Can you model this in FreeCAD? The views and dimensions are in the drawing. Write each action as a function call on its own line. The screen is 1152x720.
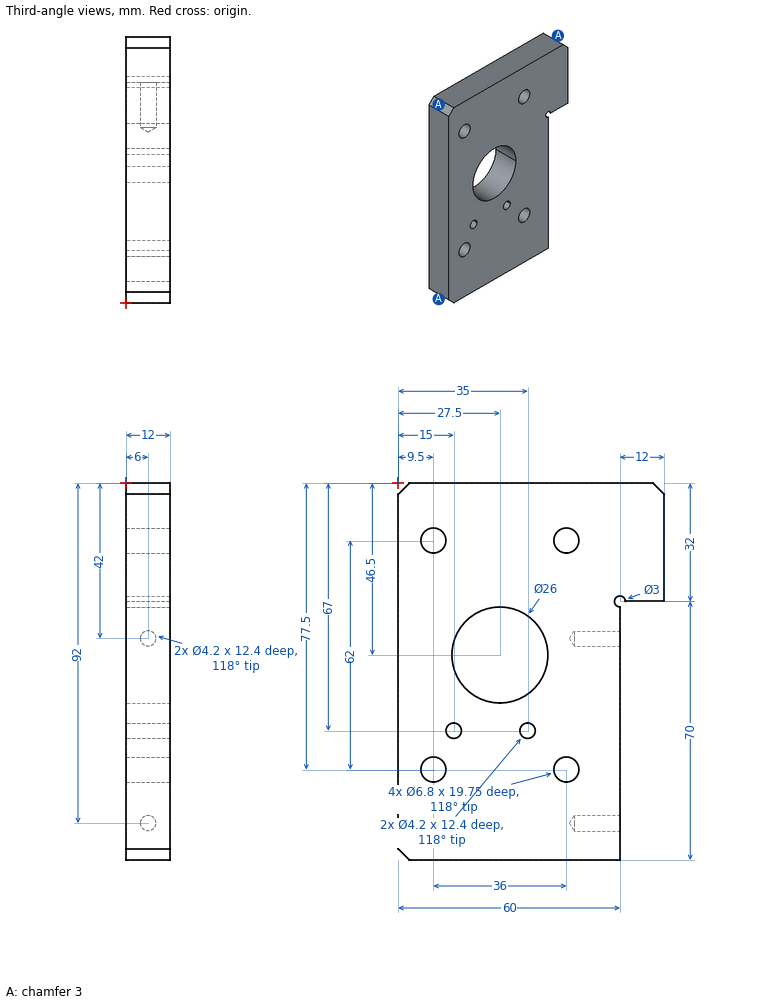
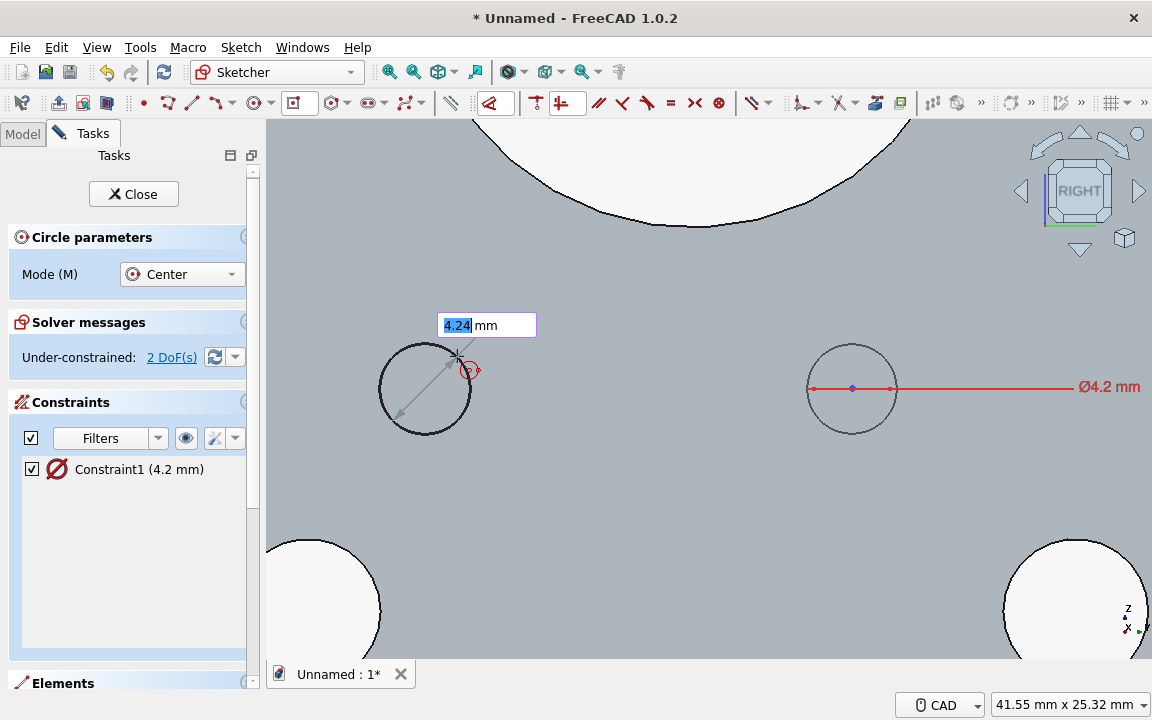
text(4.2)
key(Return)
key(Escape)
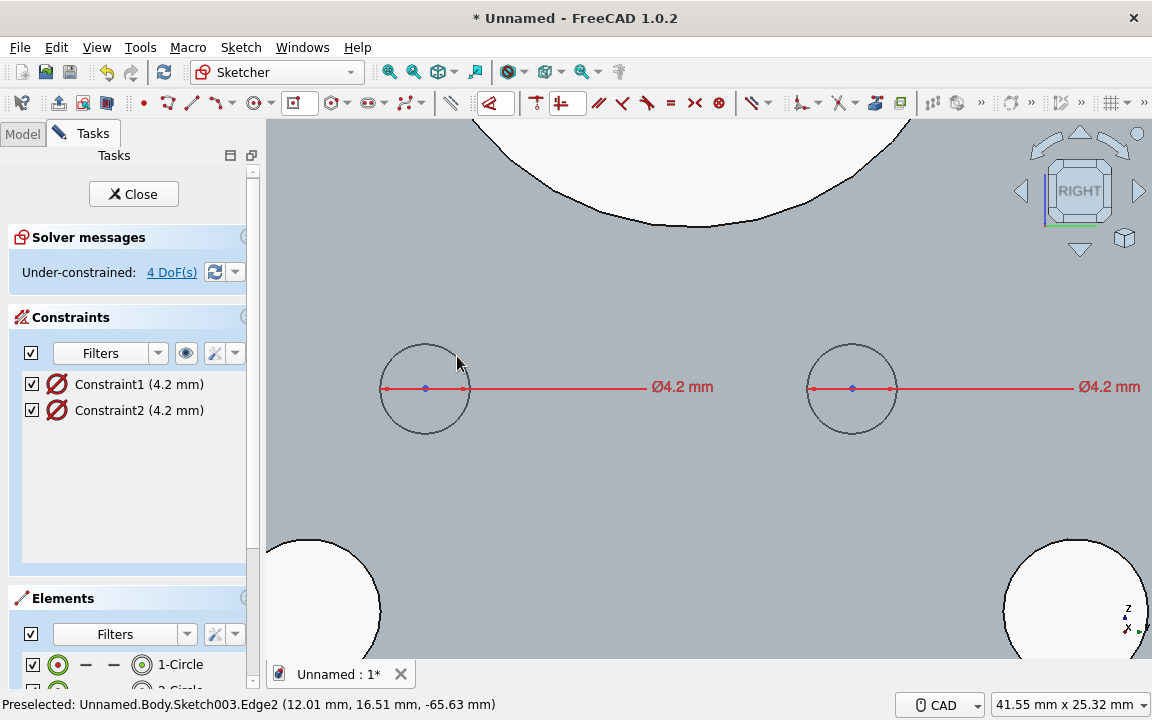
click(852, 389)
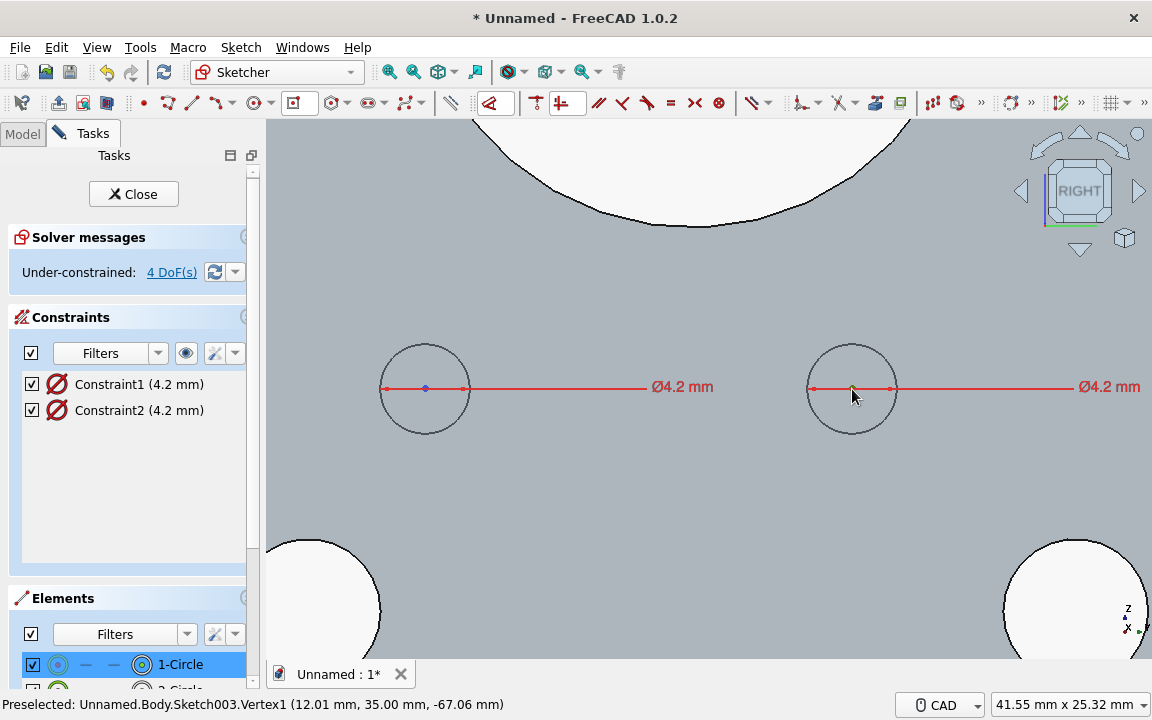
click(425, 389)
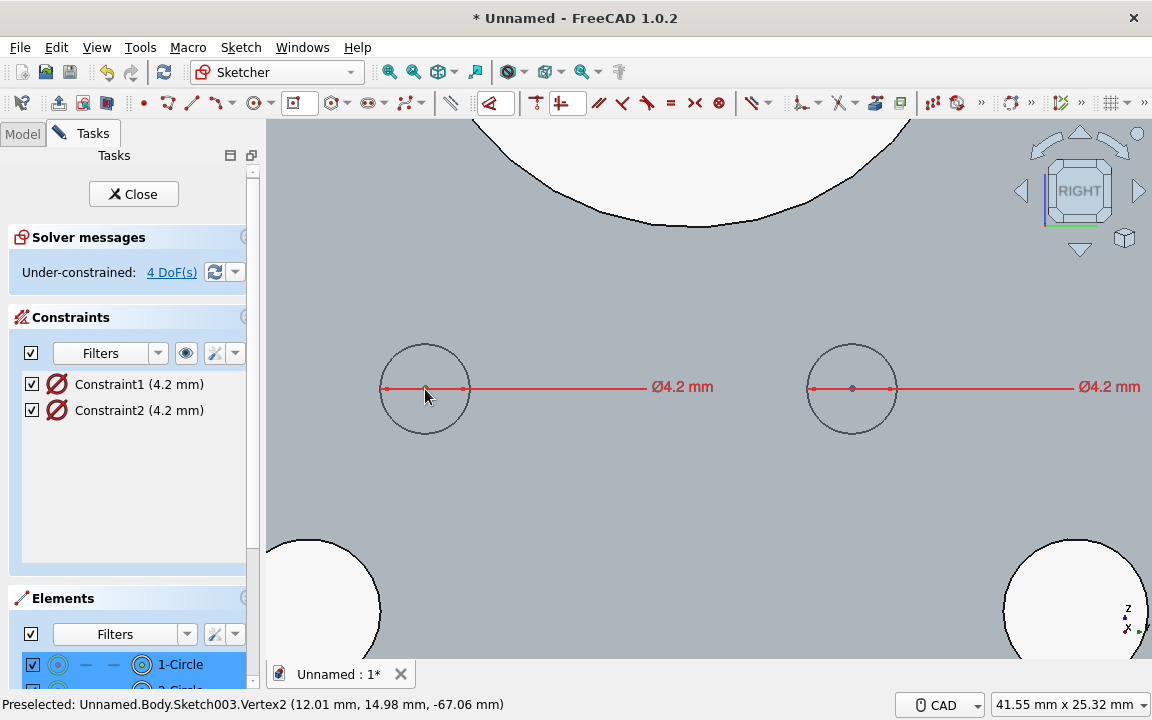
click(580, 104)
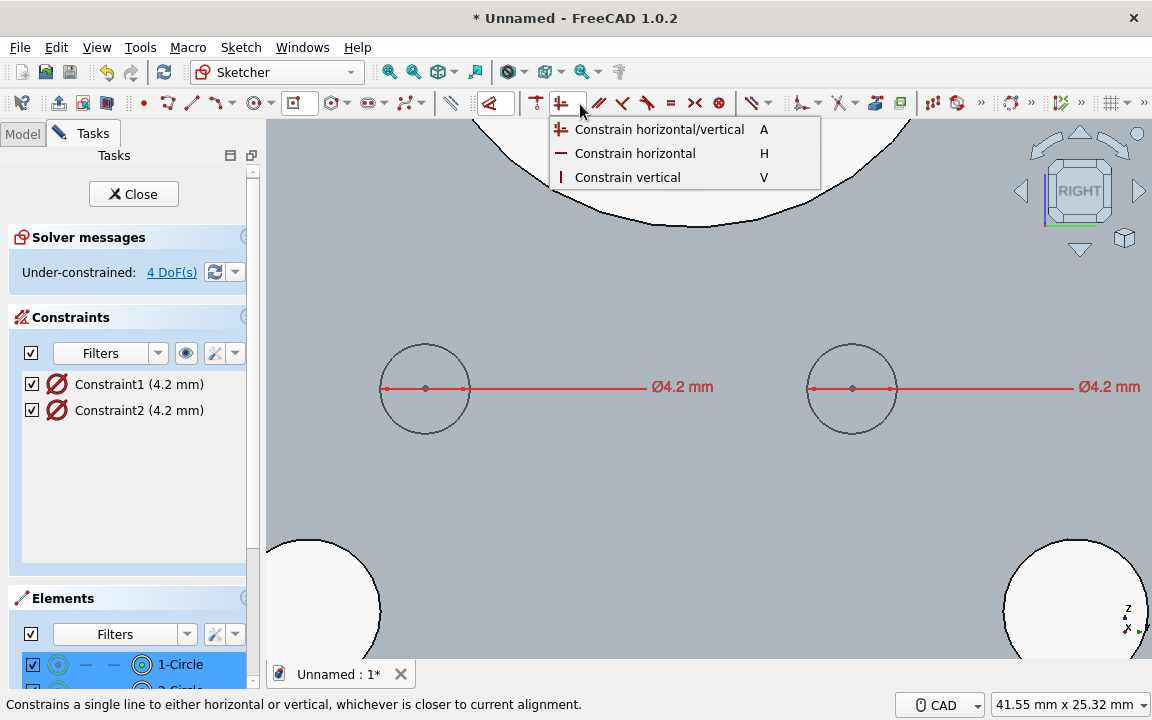
click(685, 153)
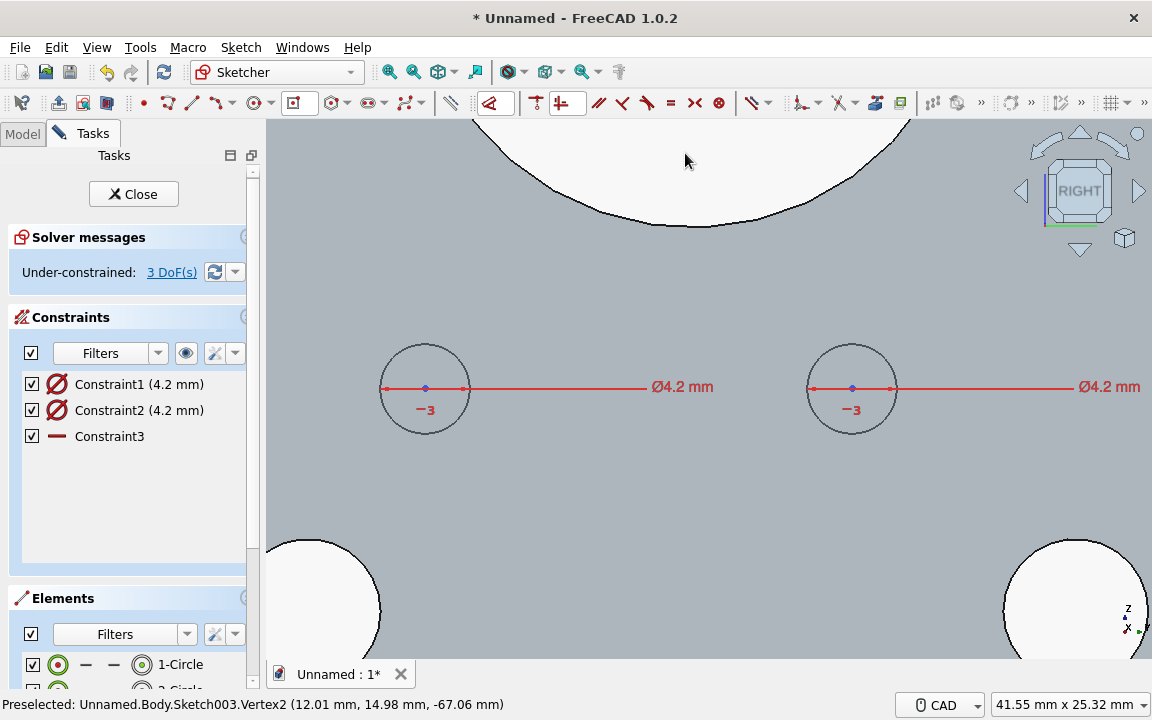
click(852, 389)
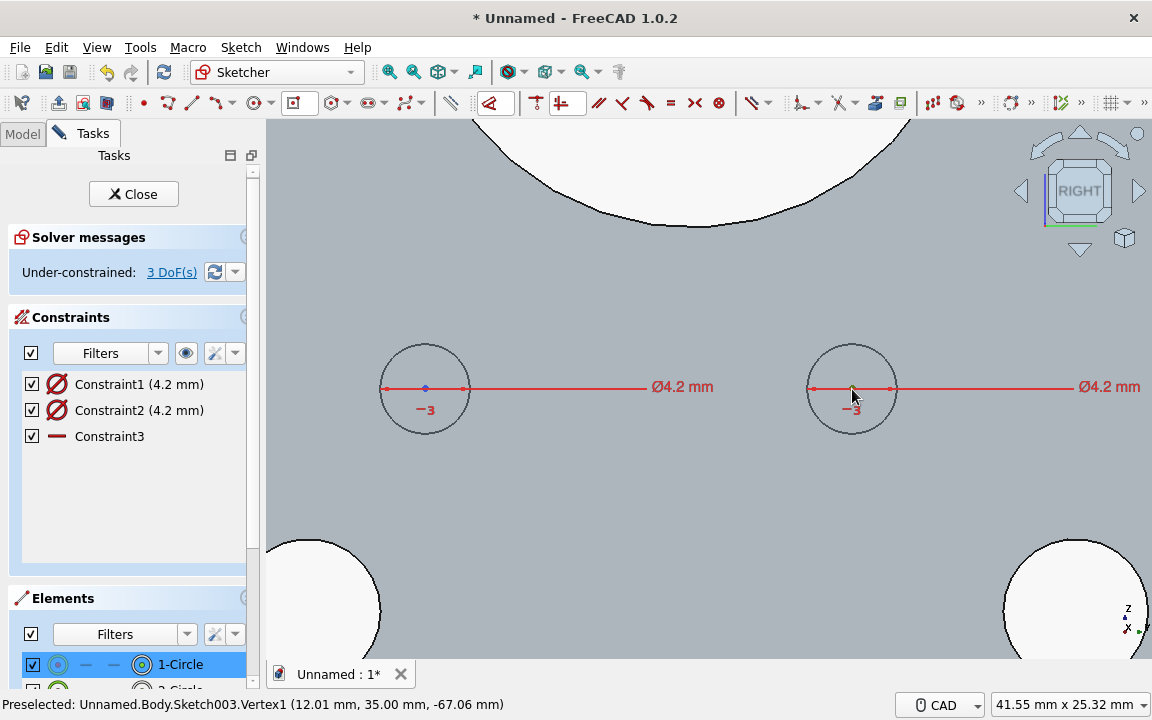
key(l)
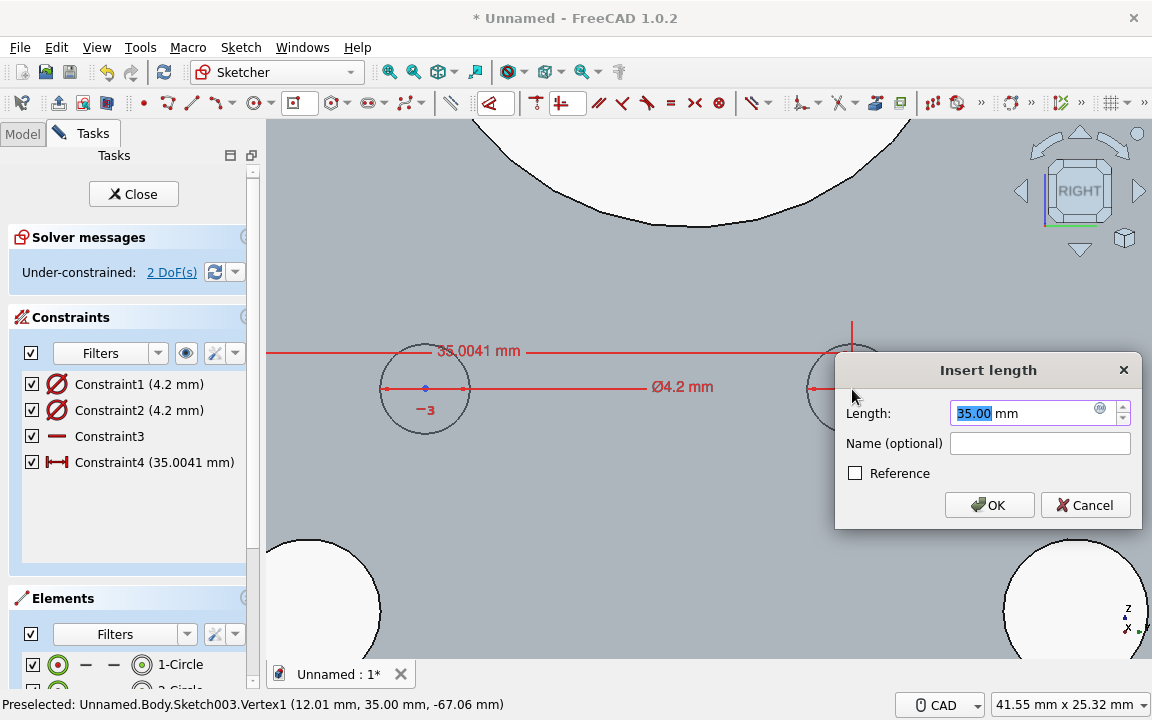
text(35)
key(Return)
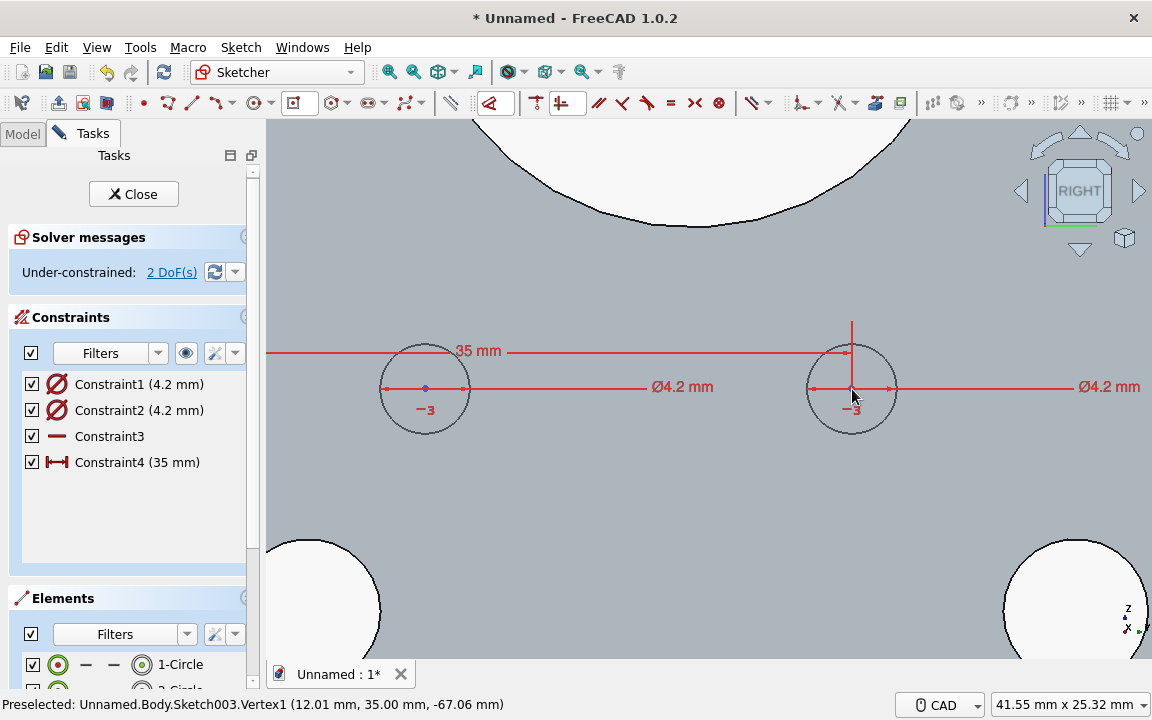
click(852, 389)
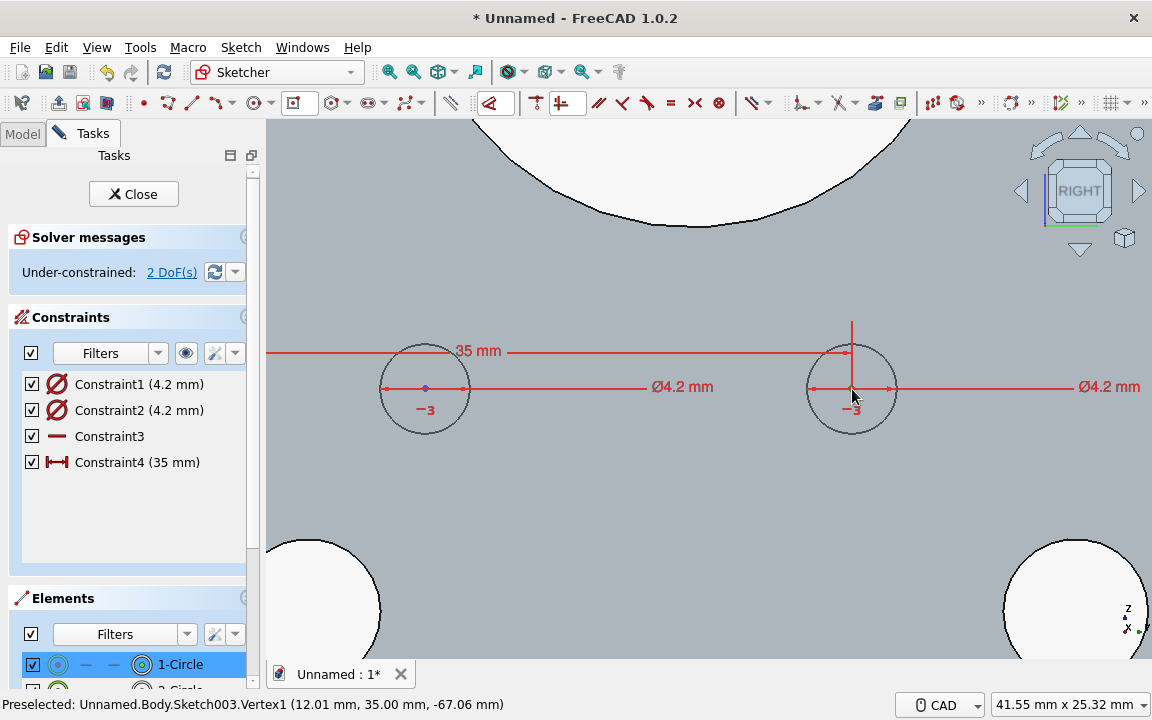
key(i)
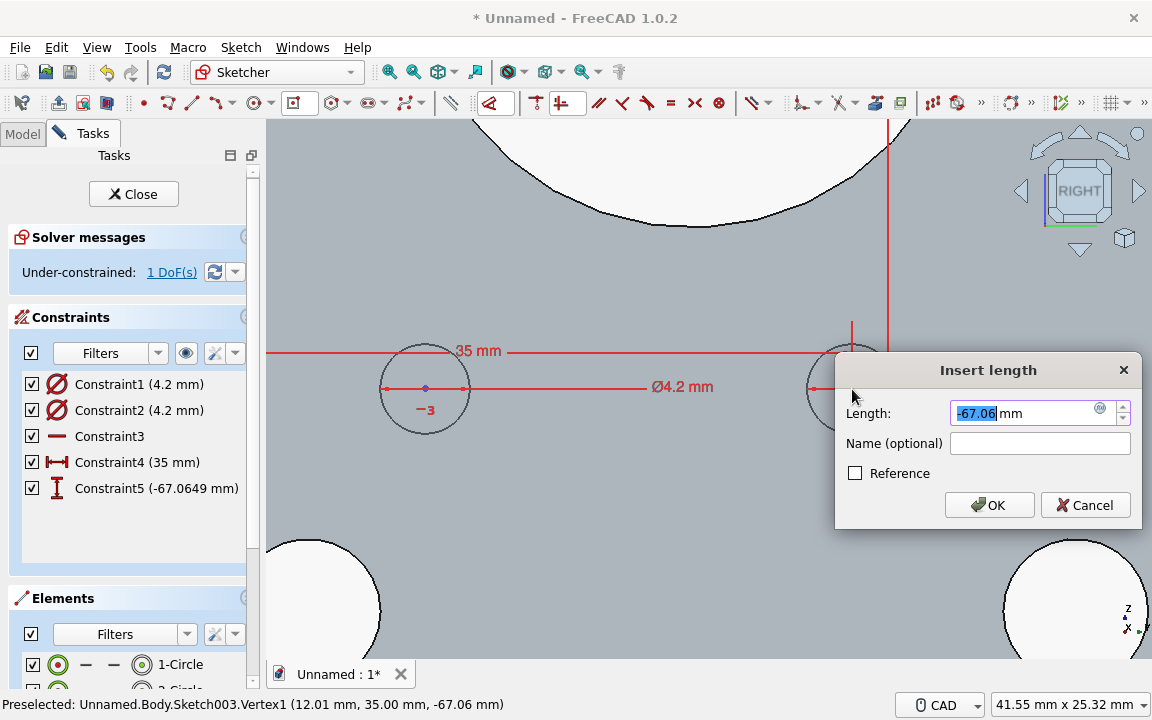
text(-67)
key(Return)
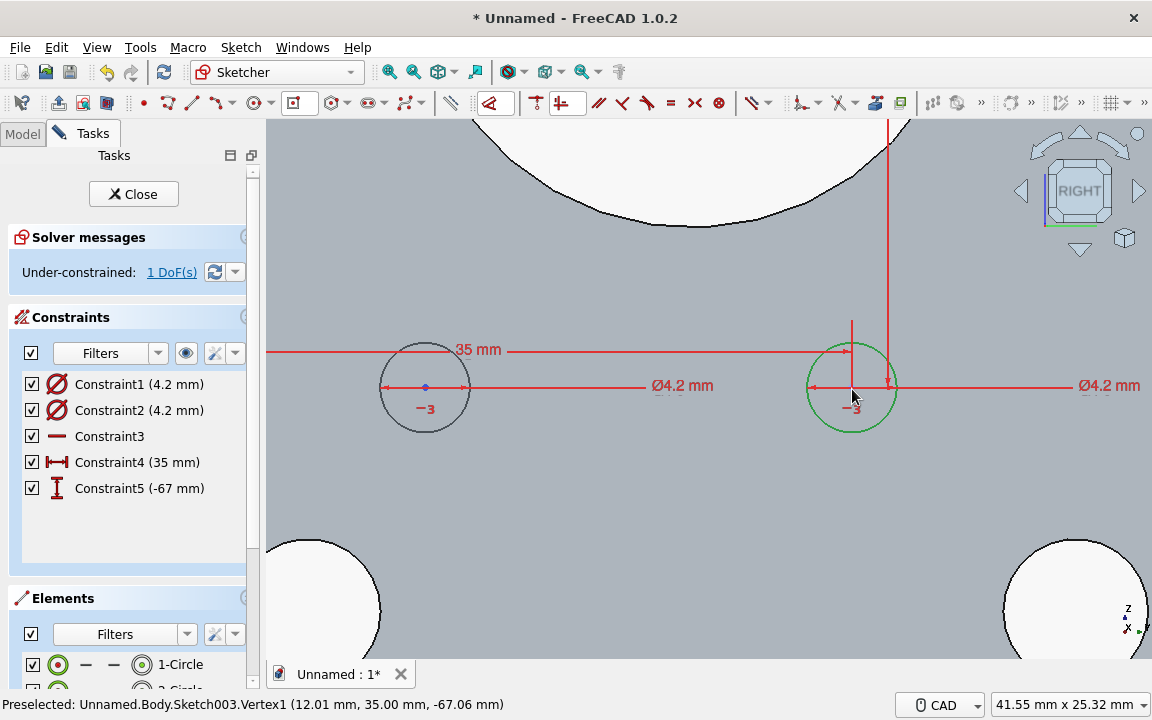
click(425, 388)